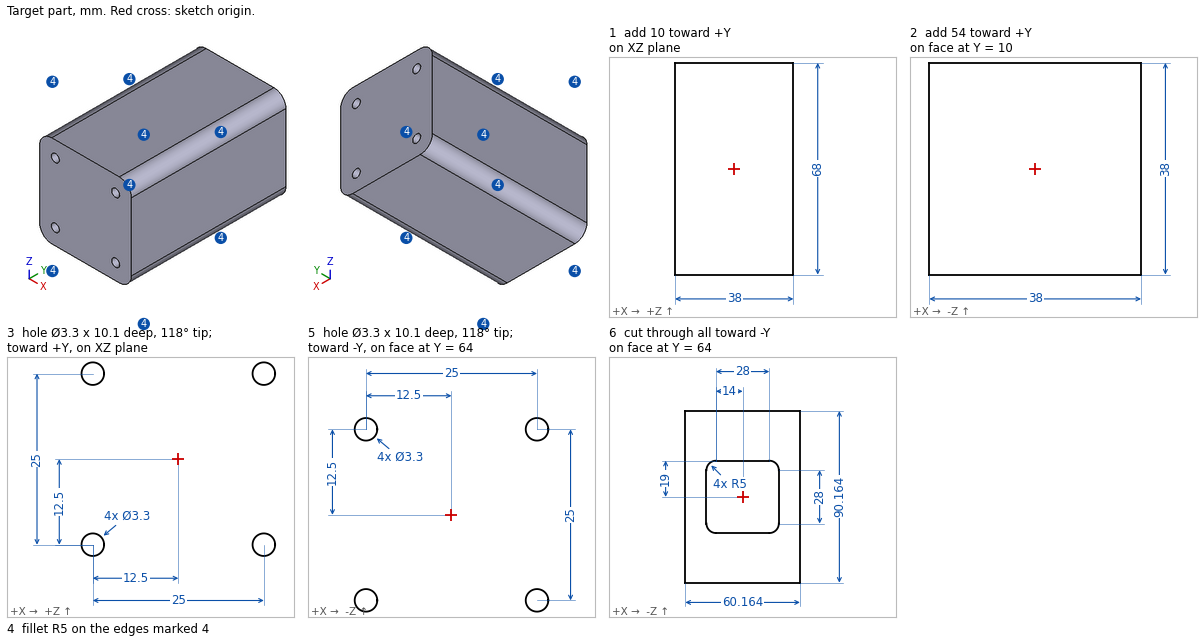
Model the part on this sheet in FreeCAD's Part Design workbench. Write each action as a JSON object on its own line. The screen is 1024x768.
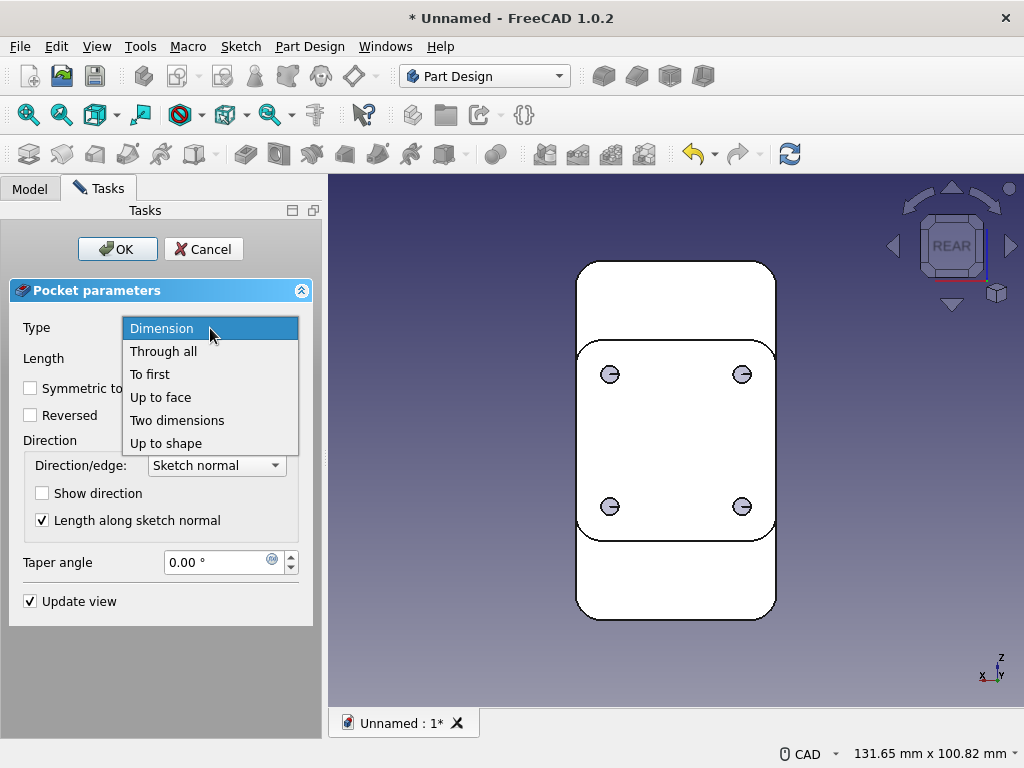
{"action": "left_click", "coordinate": [208, 352]}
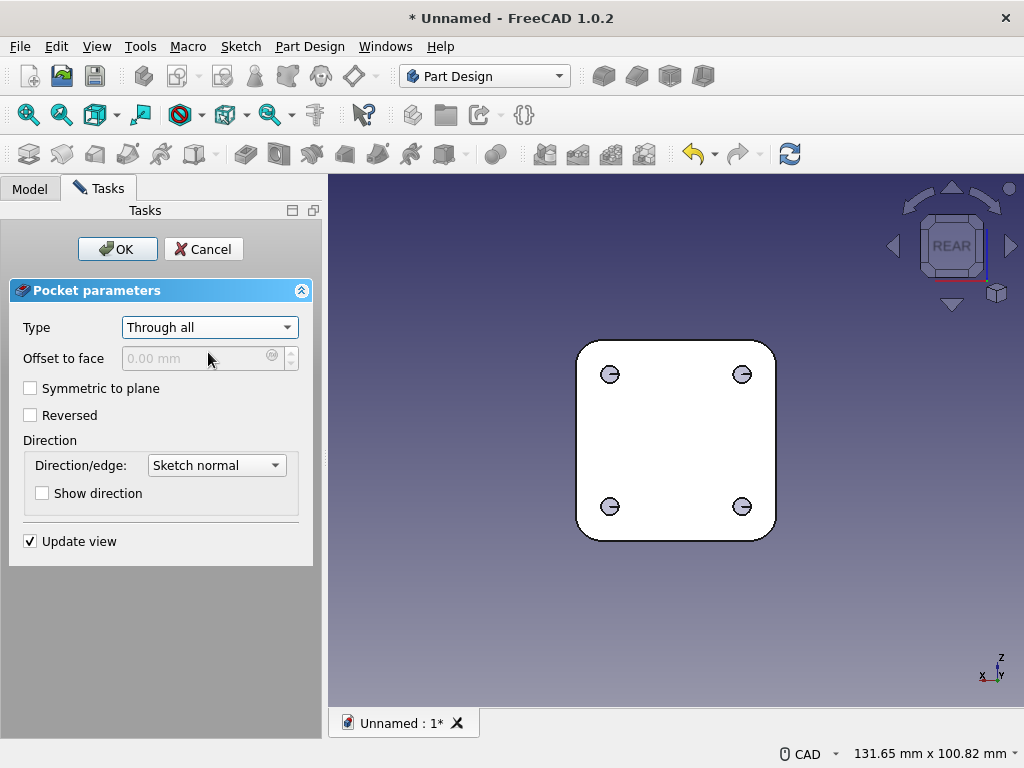
{"action": "left_click", "coordinate": [118, 249]}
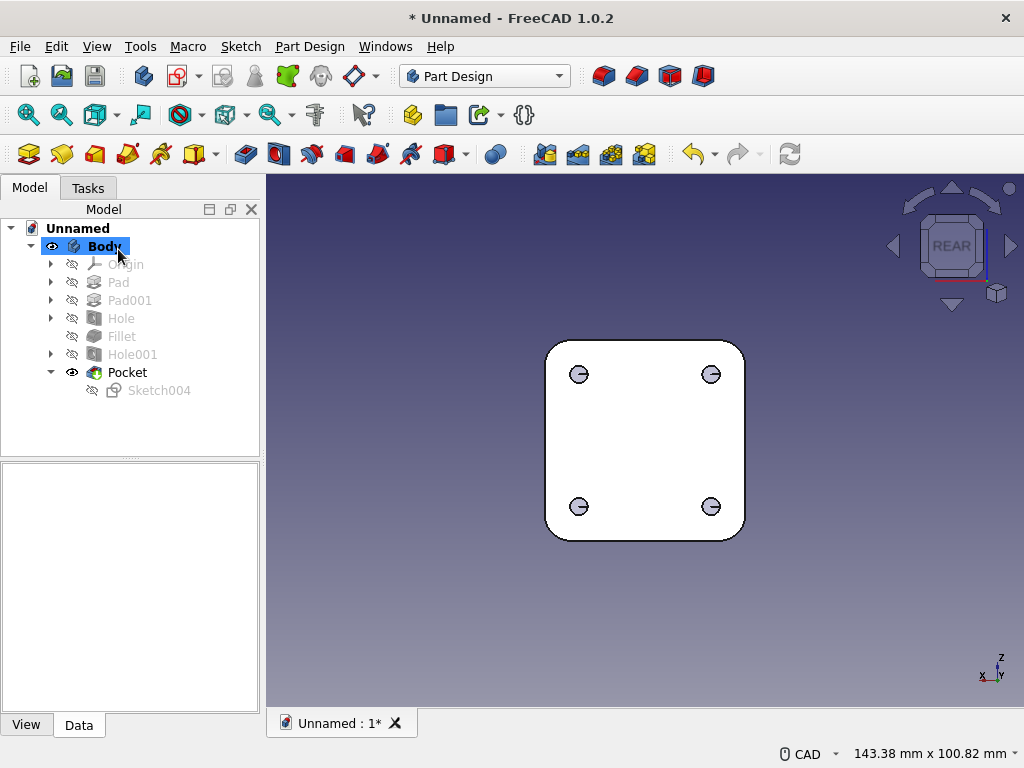
{"action": "key", "text": "0"}